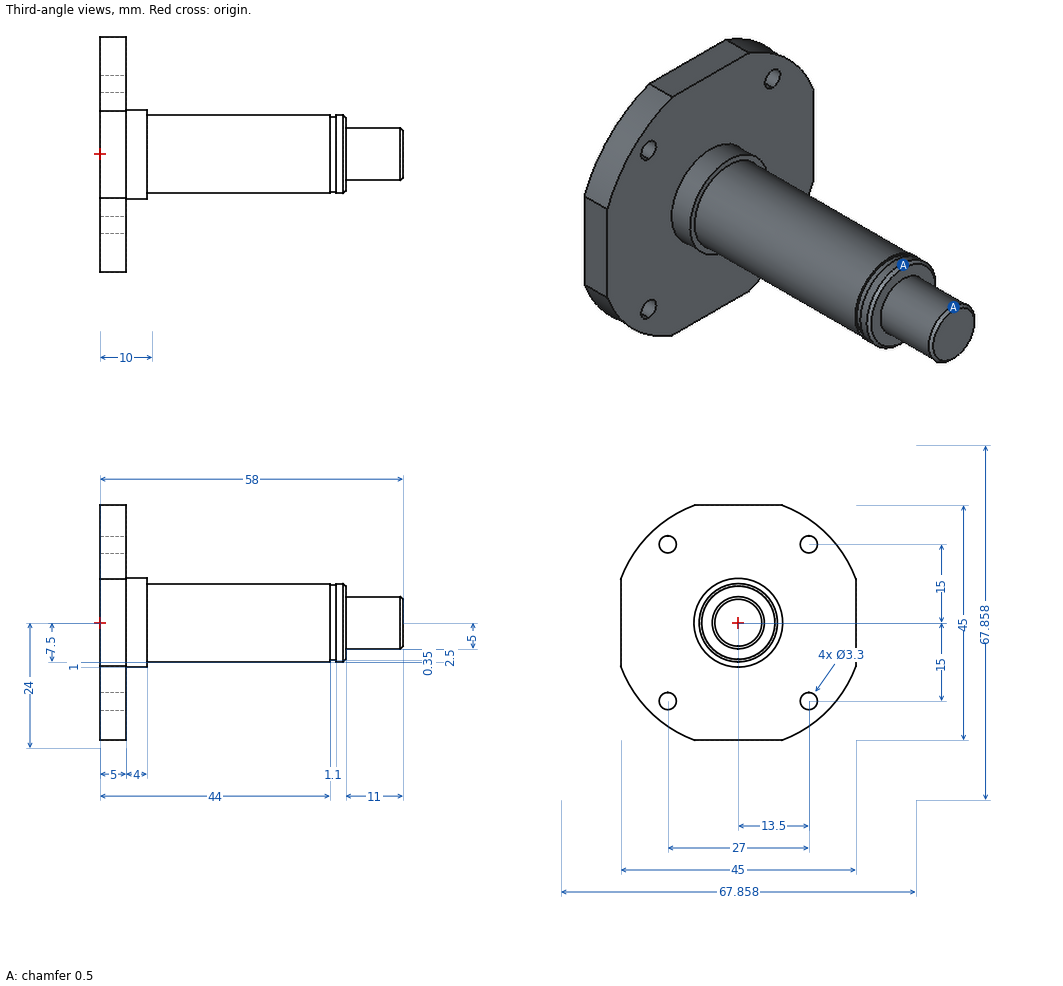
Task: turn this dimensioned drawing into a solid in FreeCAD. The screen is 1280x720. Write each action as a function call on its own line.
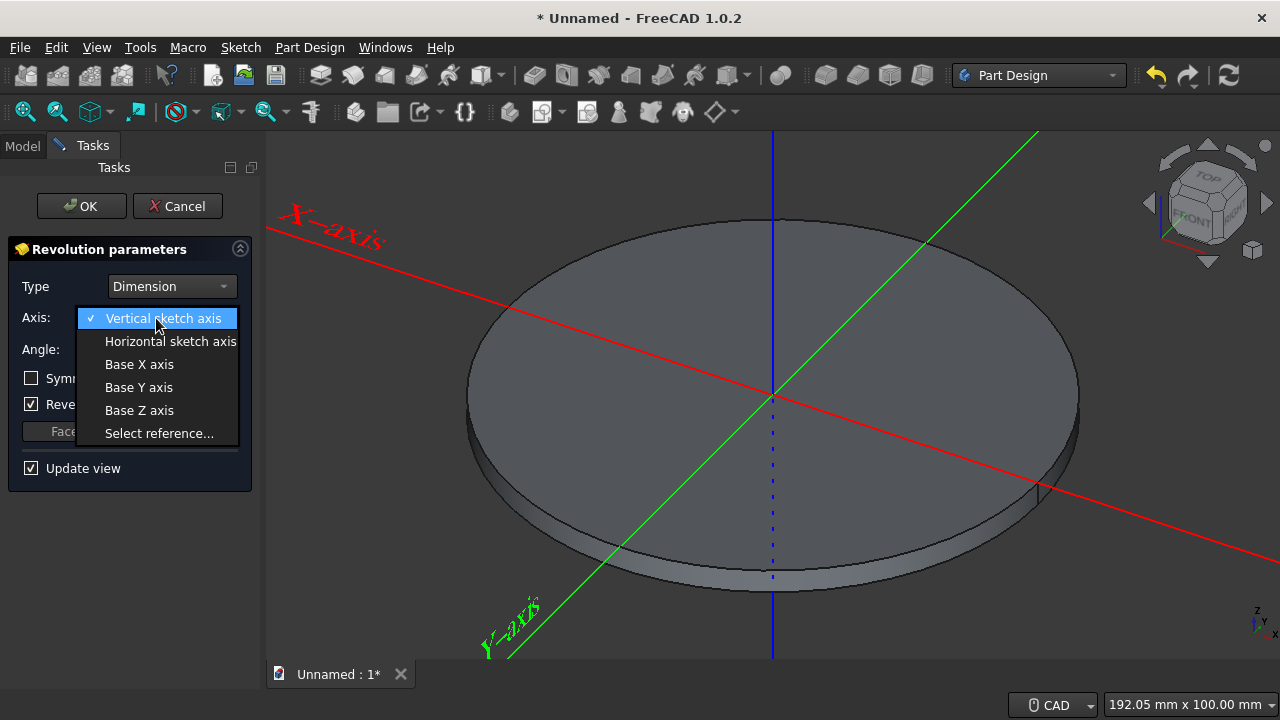
click(156, 342)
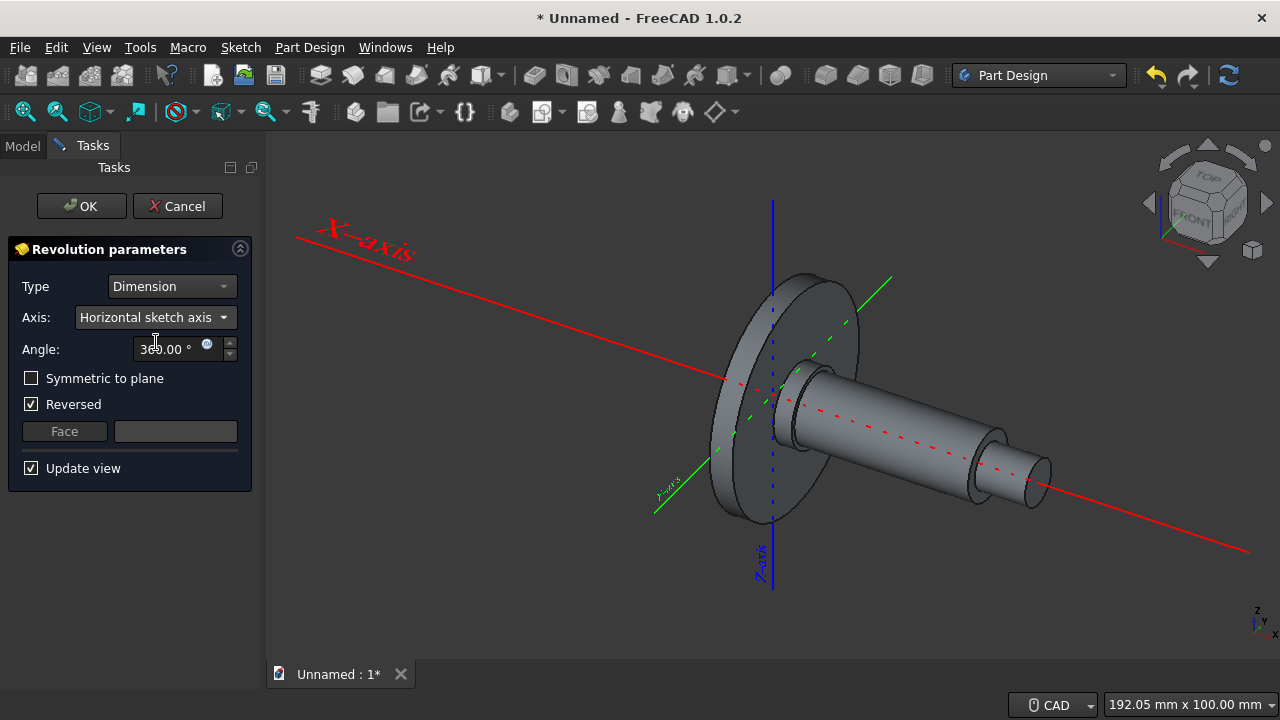
click(82, 206)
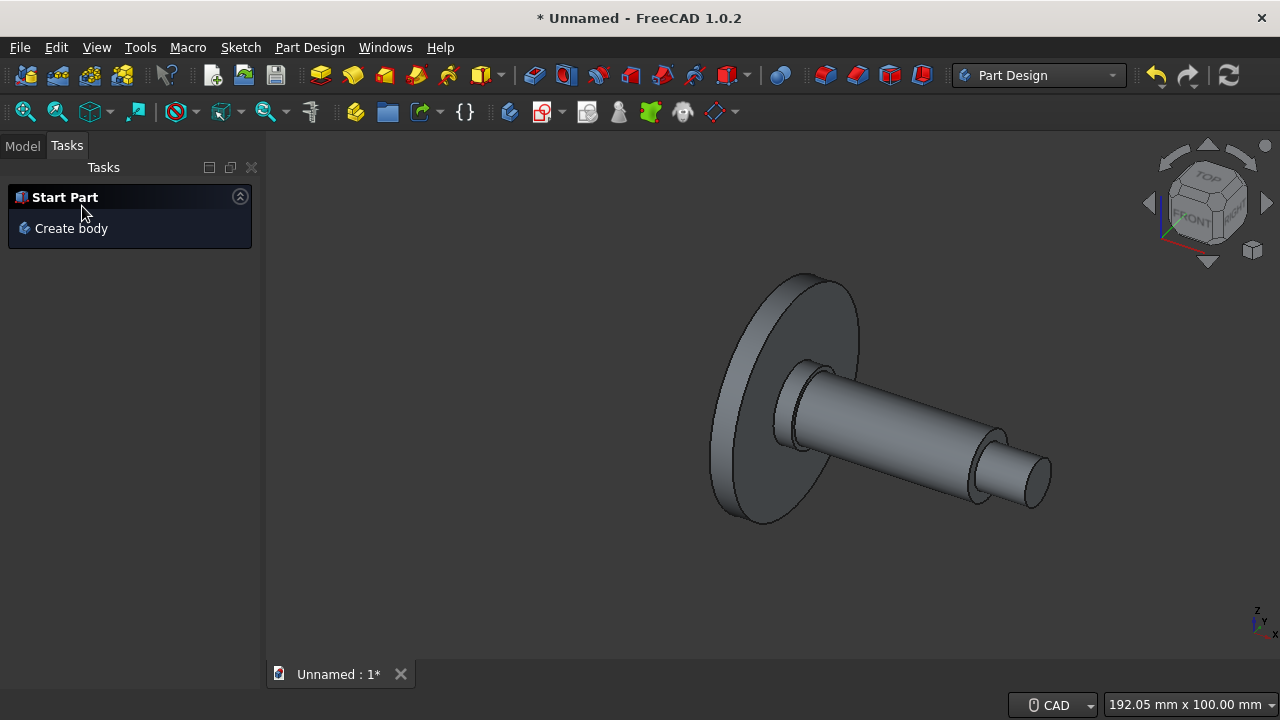
key(6)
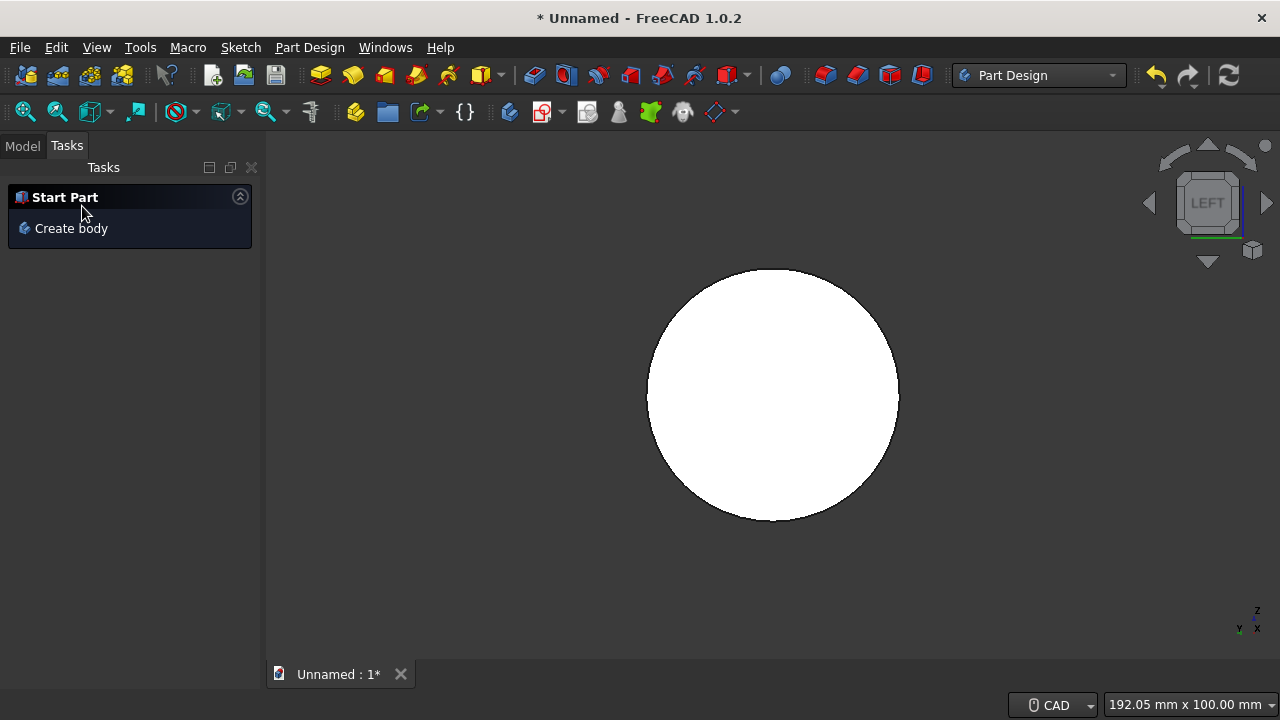
click(773, 394)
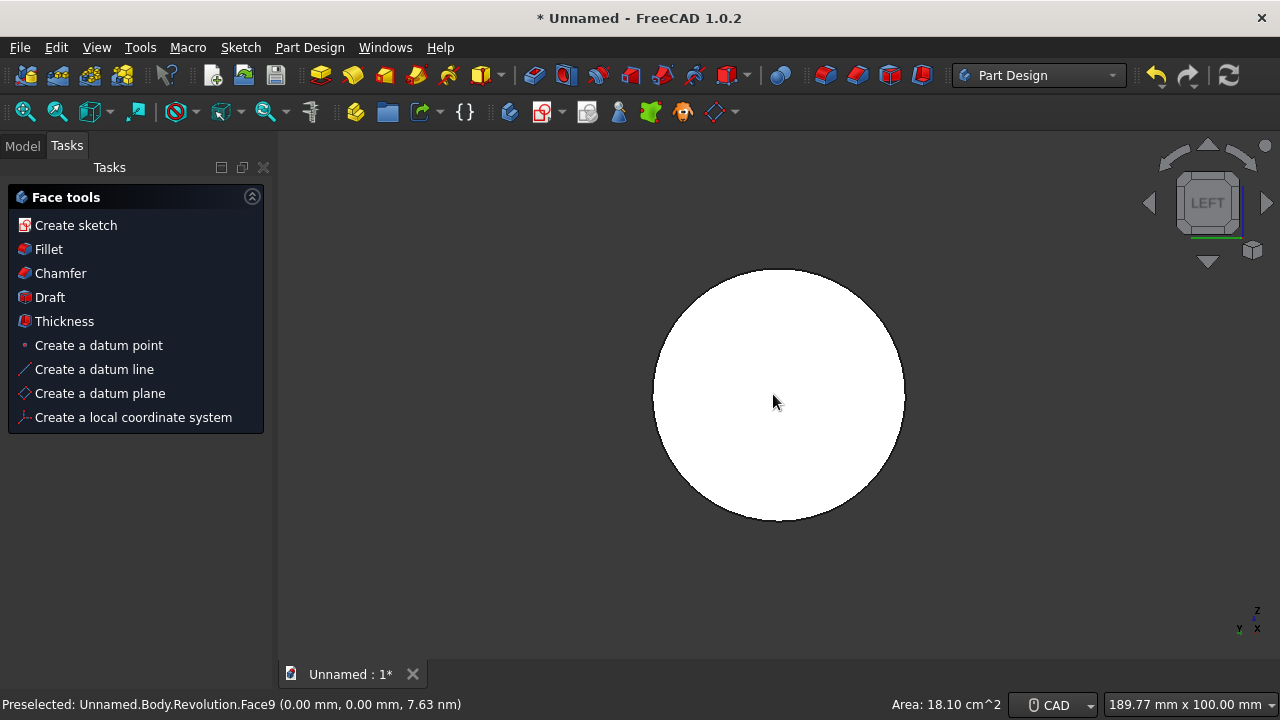
click(542, 112)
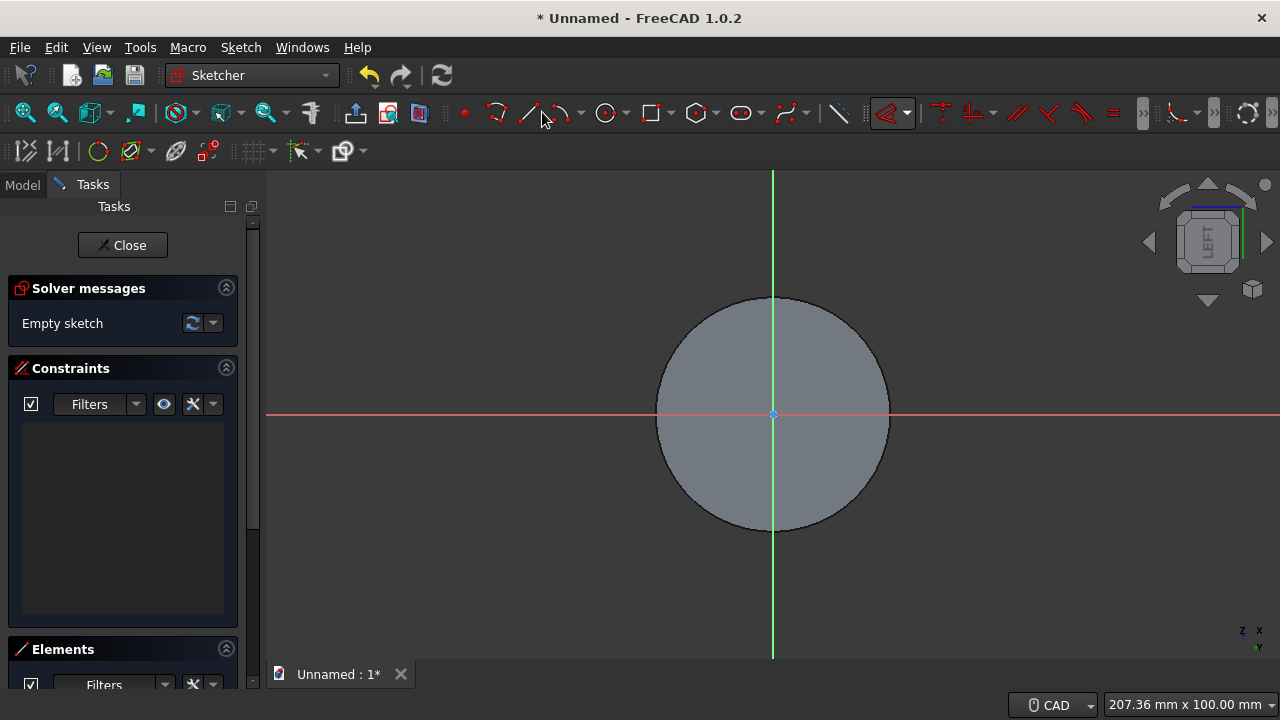
scroll(829, 414, up, 4)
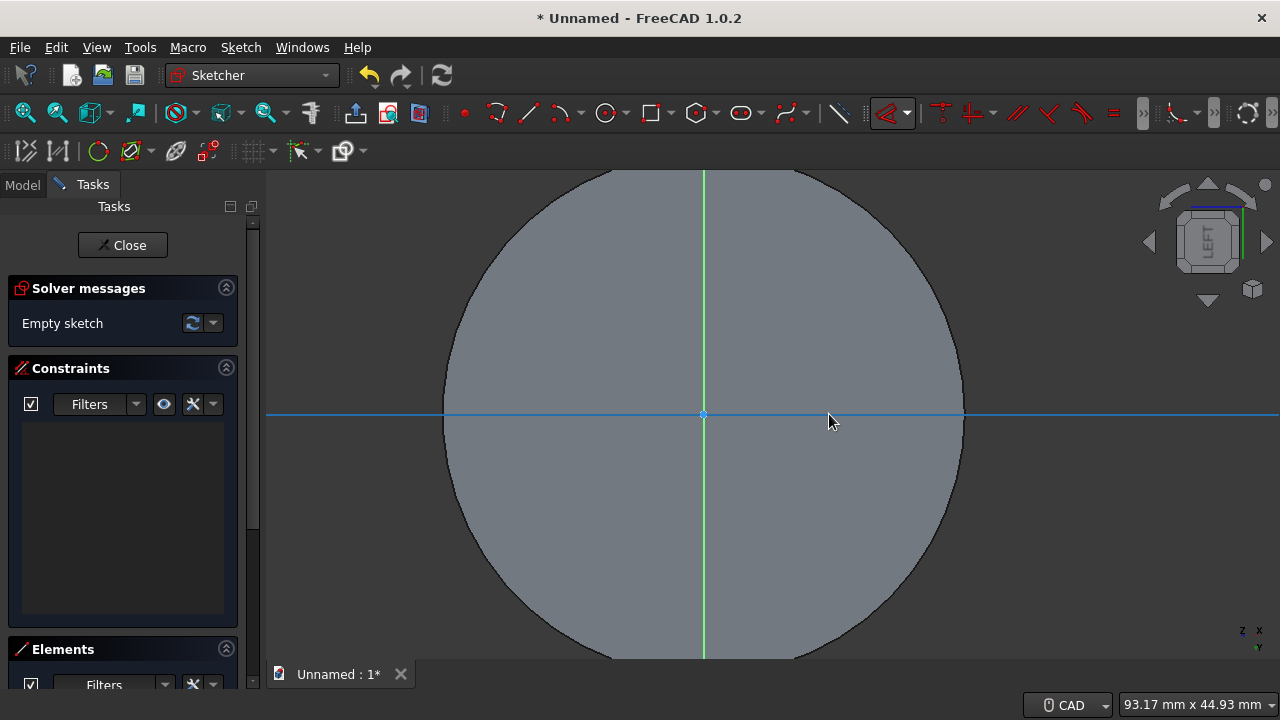
click(606, 114)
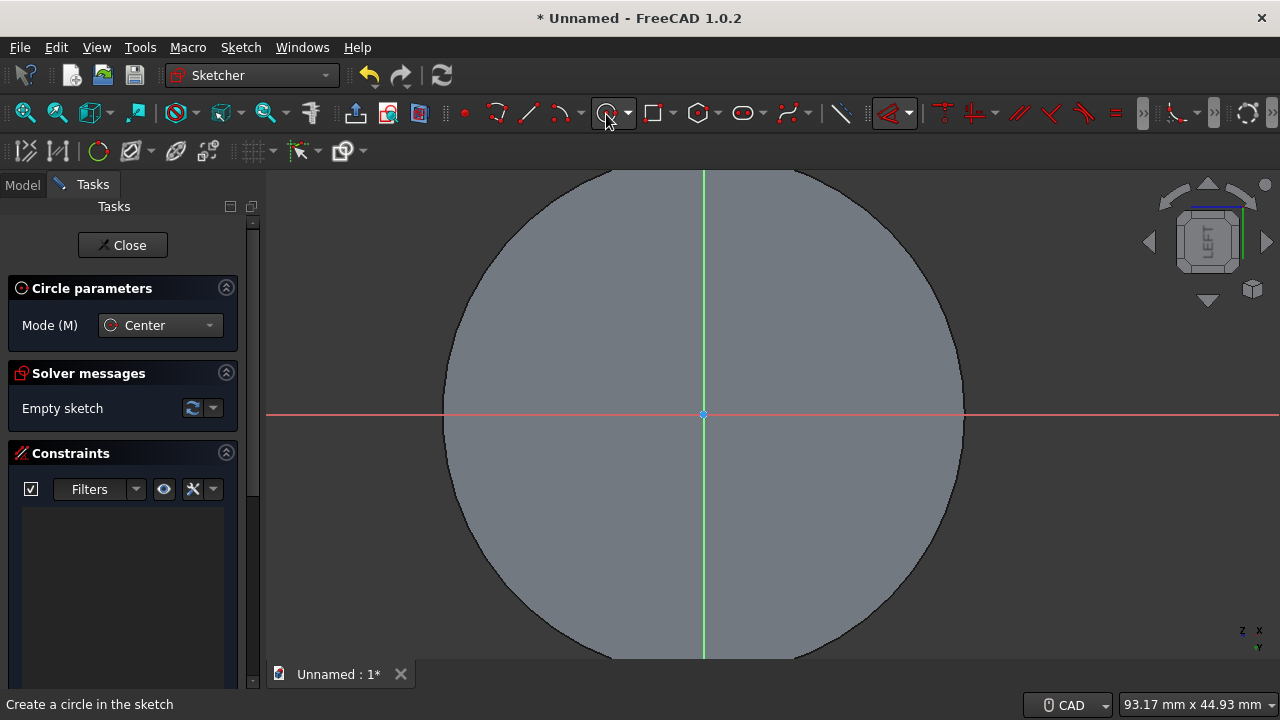
scroll(867, 561, up, 2)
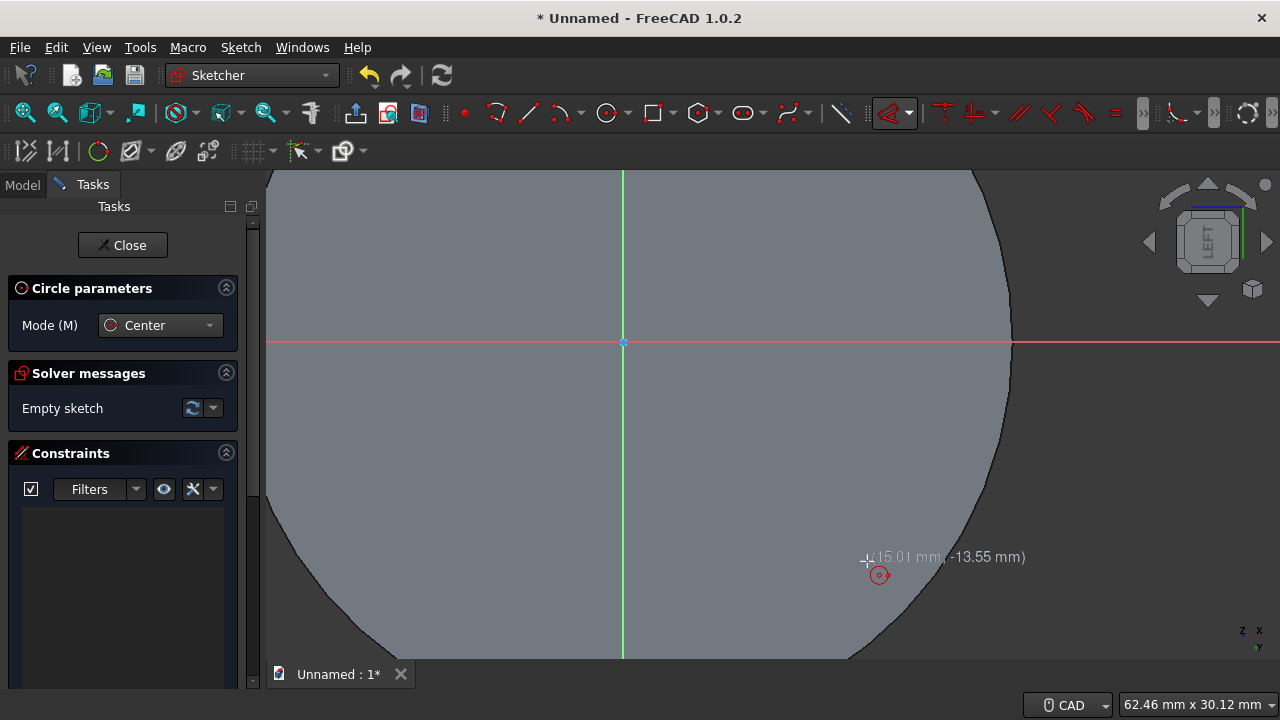
click(867, 561)
click(886, 542)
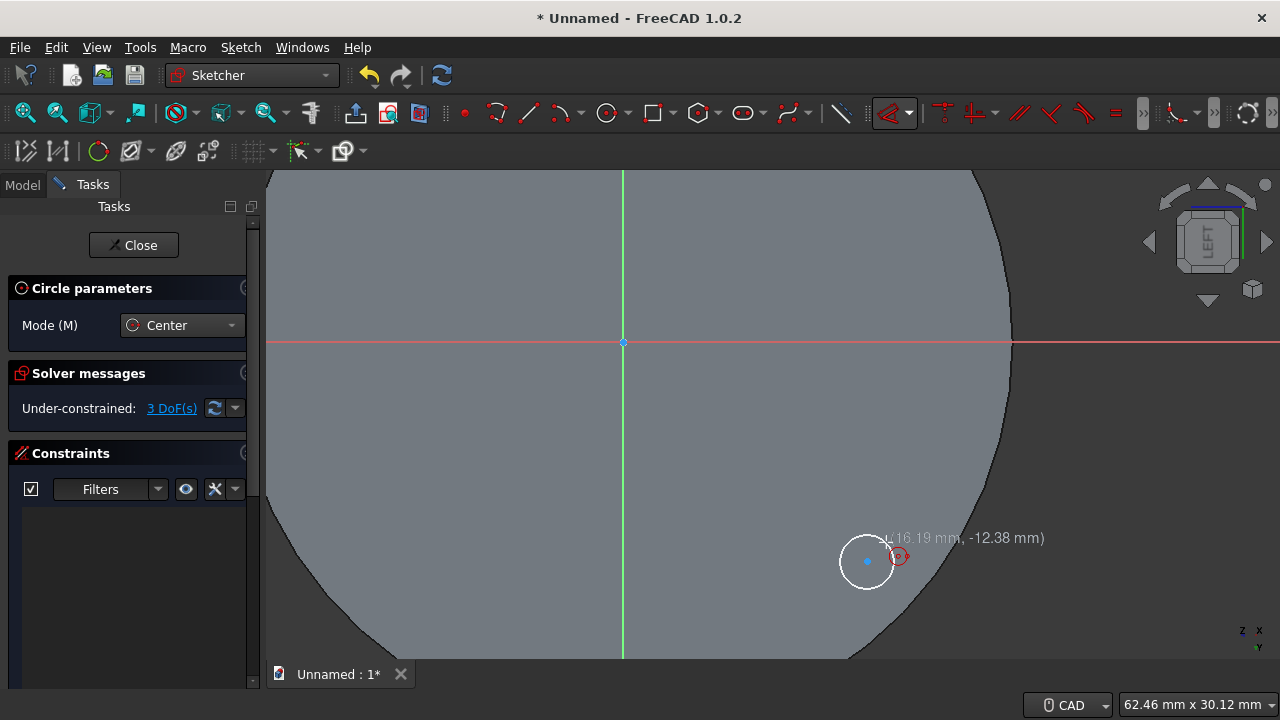
click(380, 561)
click(398, 542)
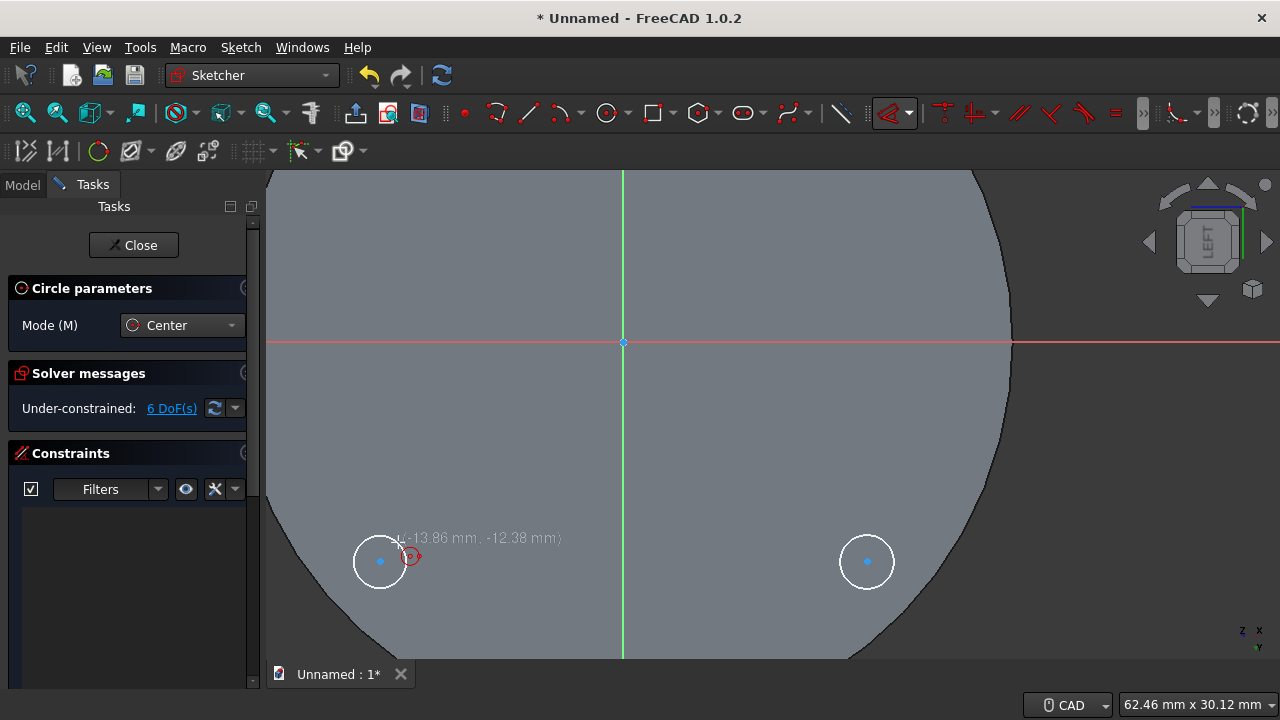
scroll(870, 562, down, 2)